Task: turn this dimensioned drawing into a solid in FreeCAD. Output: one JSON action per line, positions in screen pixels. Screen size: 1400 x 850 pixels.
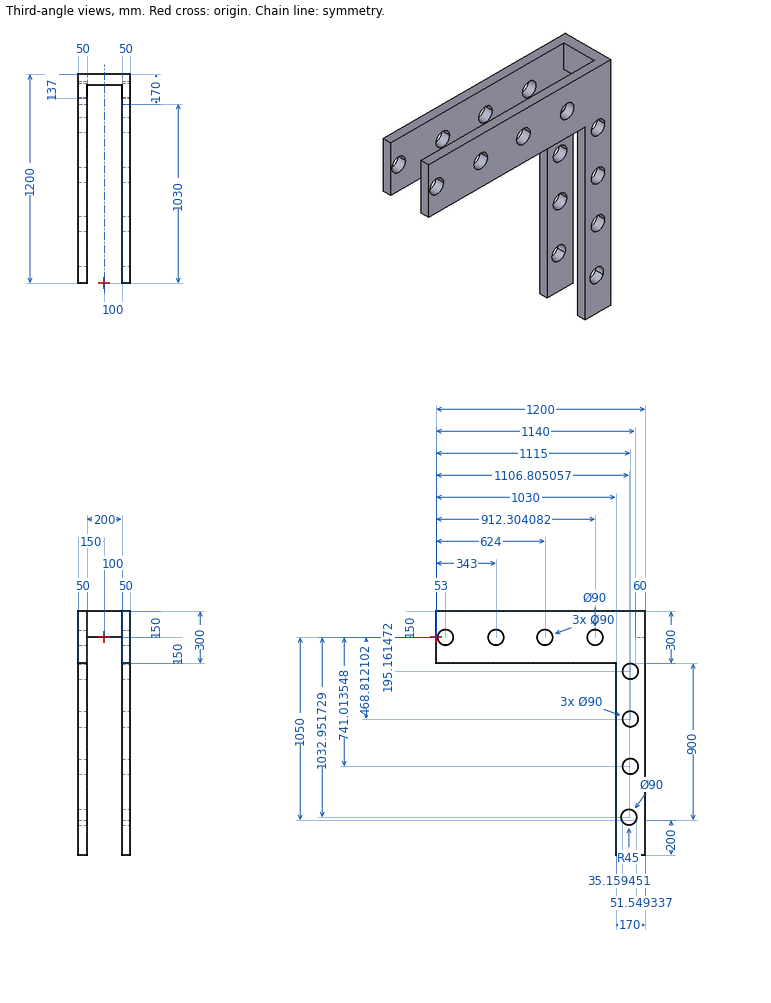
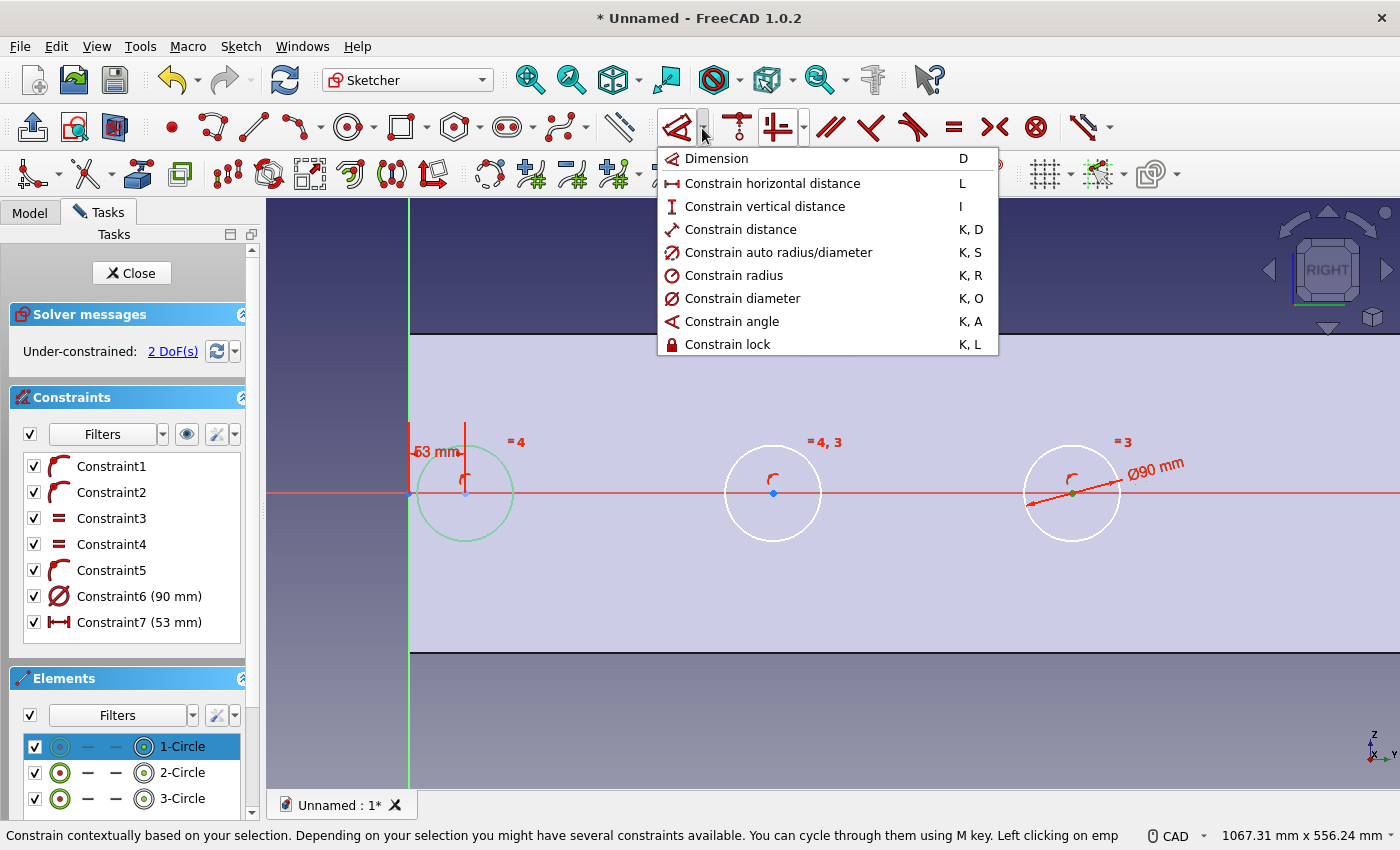
{"action": "left_click", "coordinate": [828, 184]}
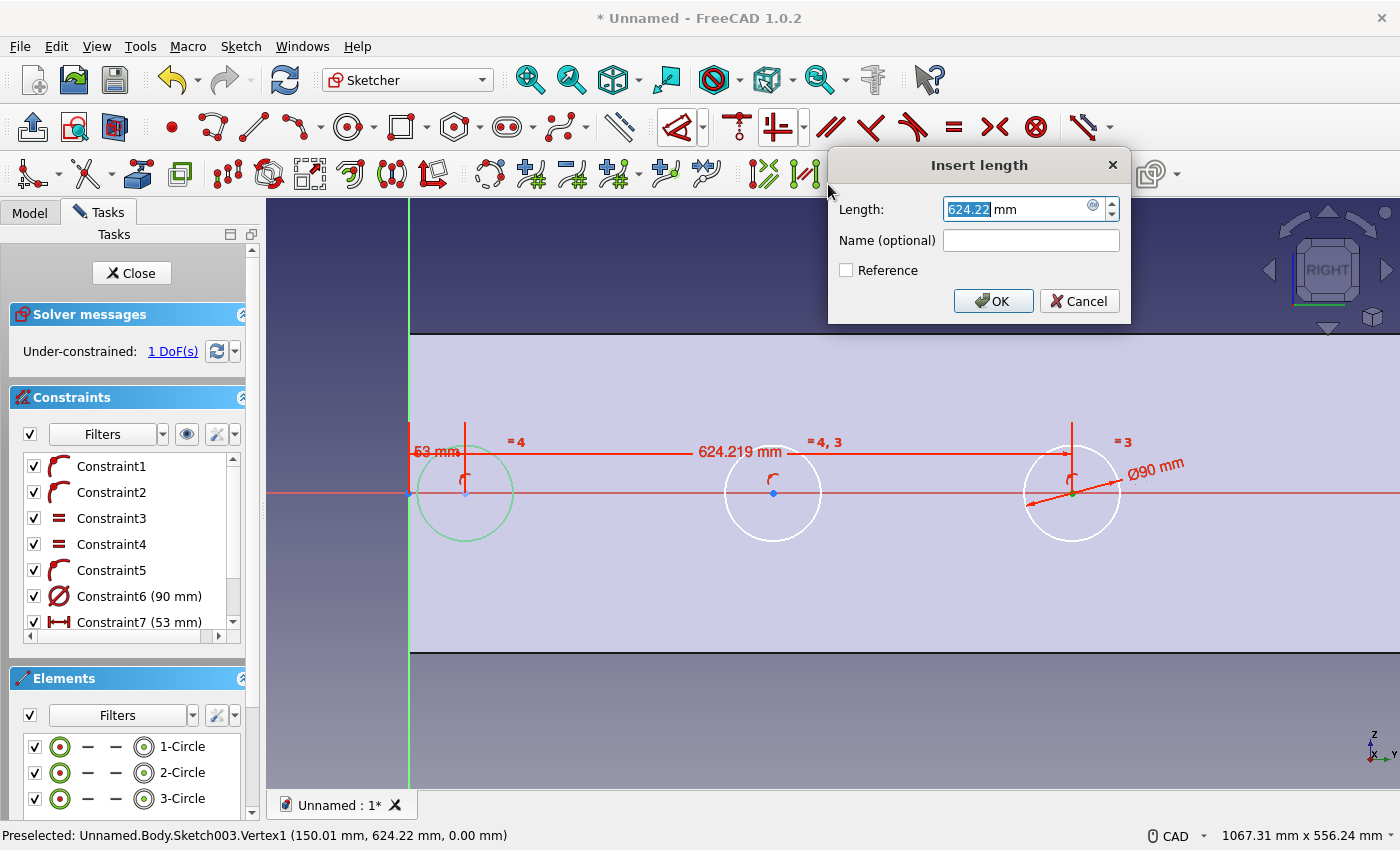
{"action": "type", "text": "624"}
{"action": "key", "text": "Return"}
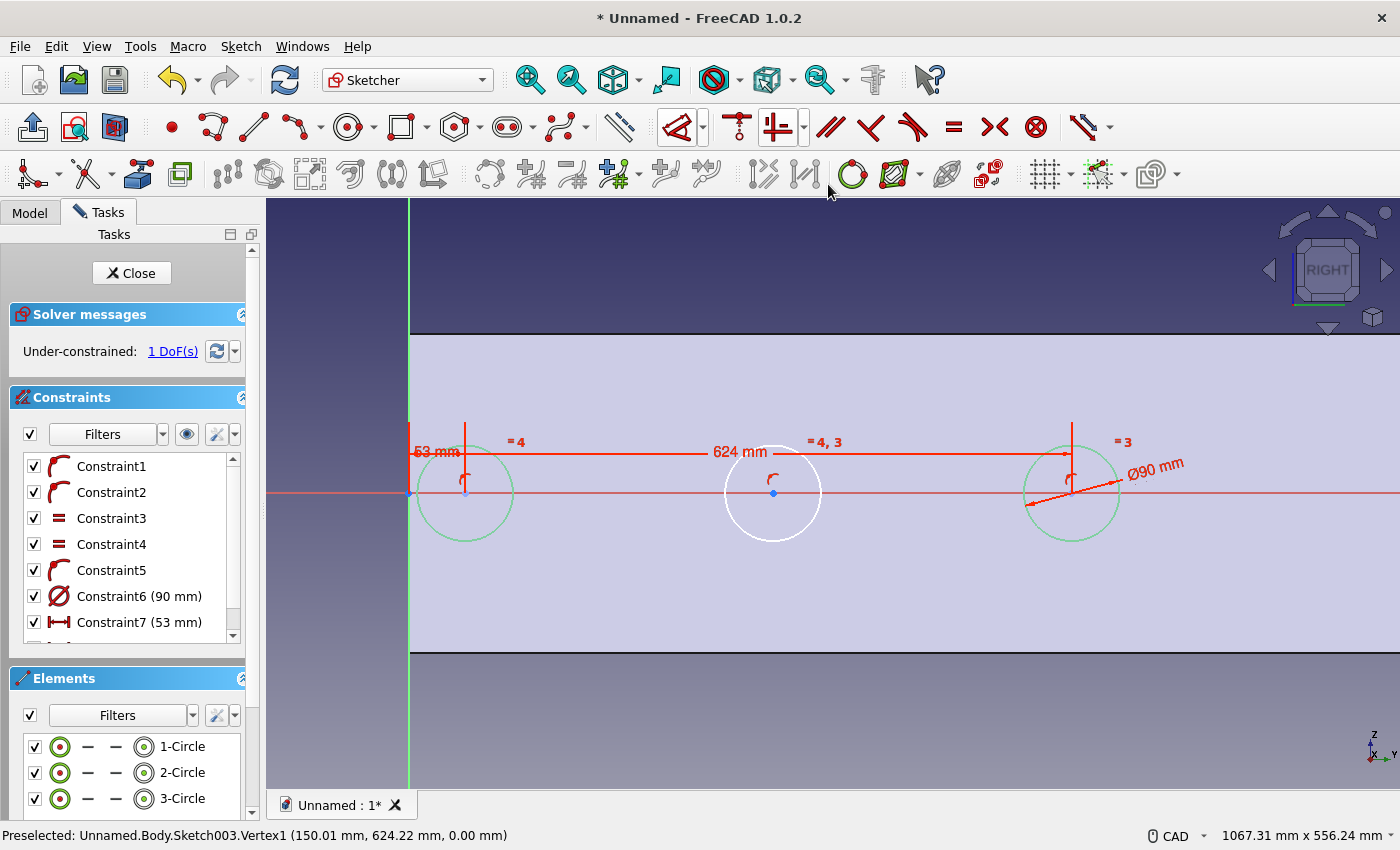
{"action": "left_click", "coordinate": [773, 493]}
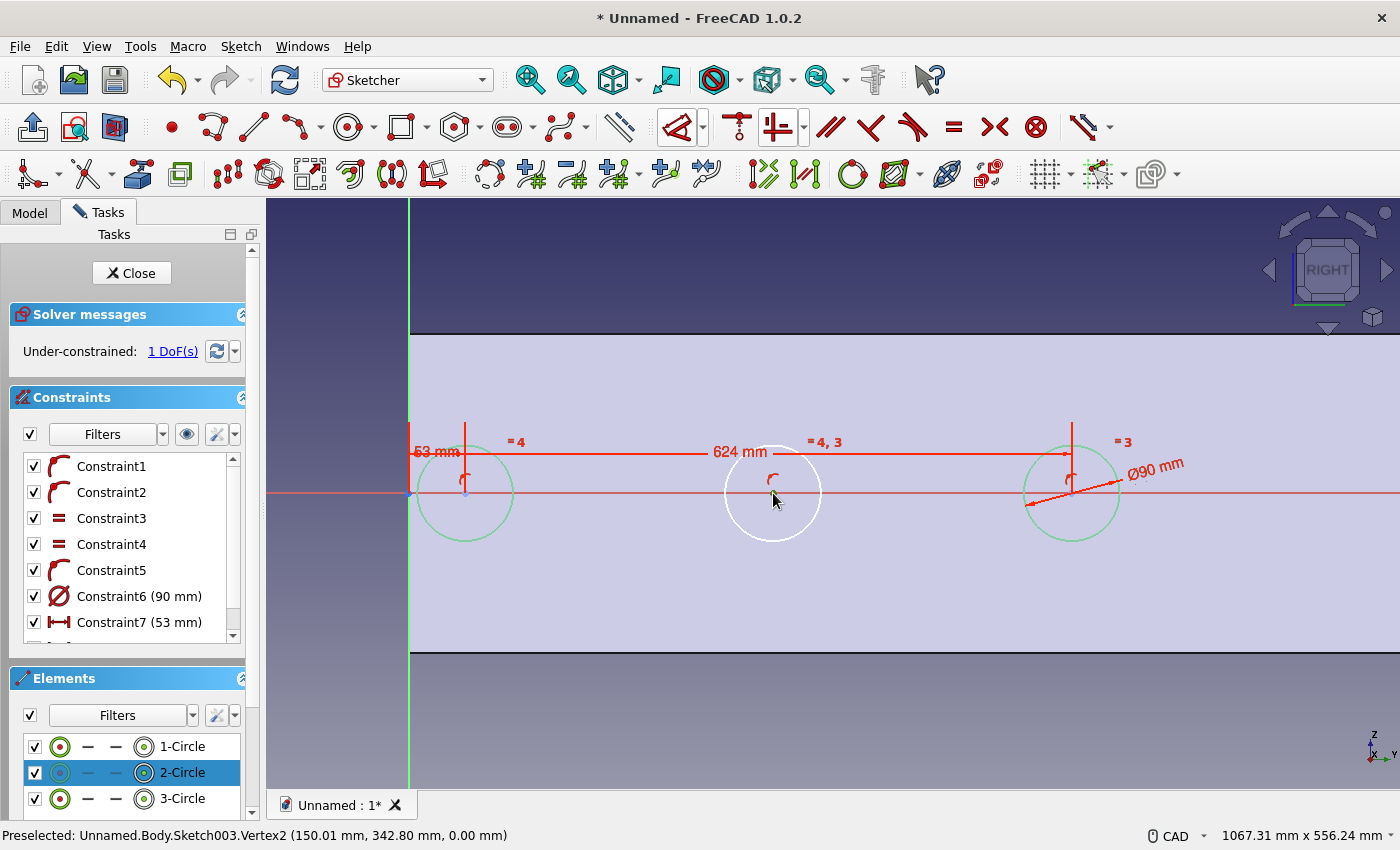
{"action": "left_click", "coordinate": [702, 128]}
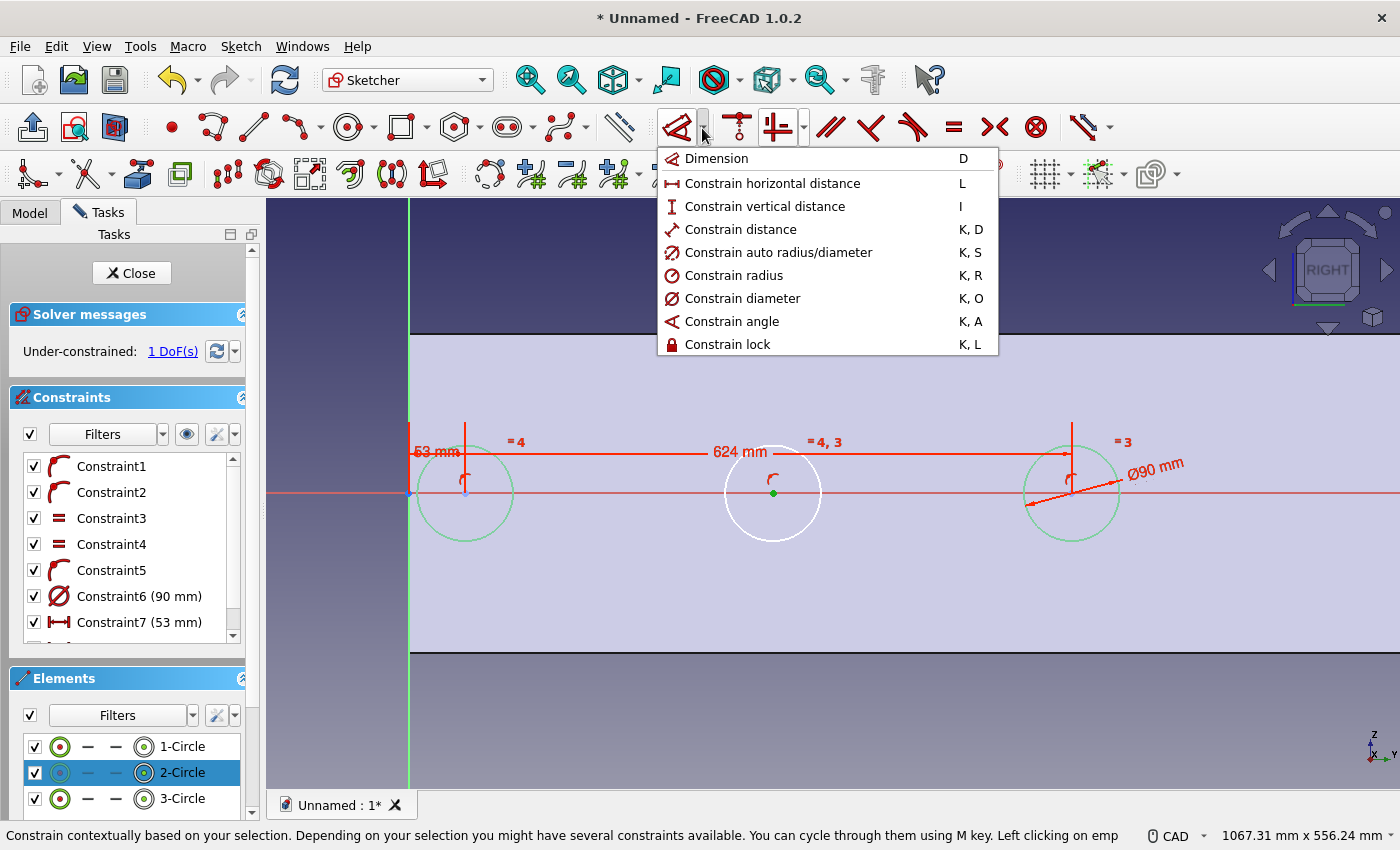
{"action": "left_click", "coordinate": [828, 184]}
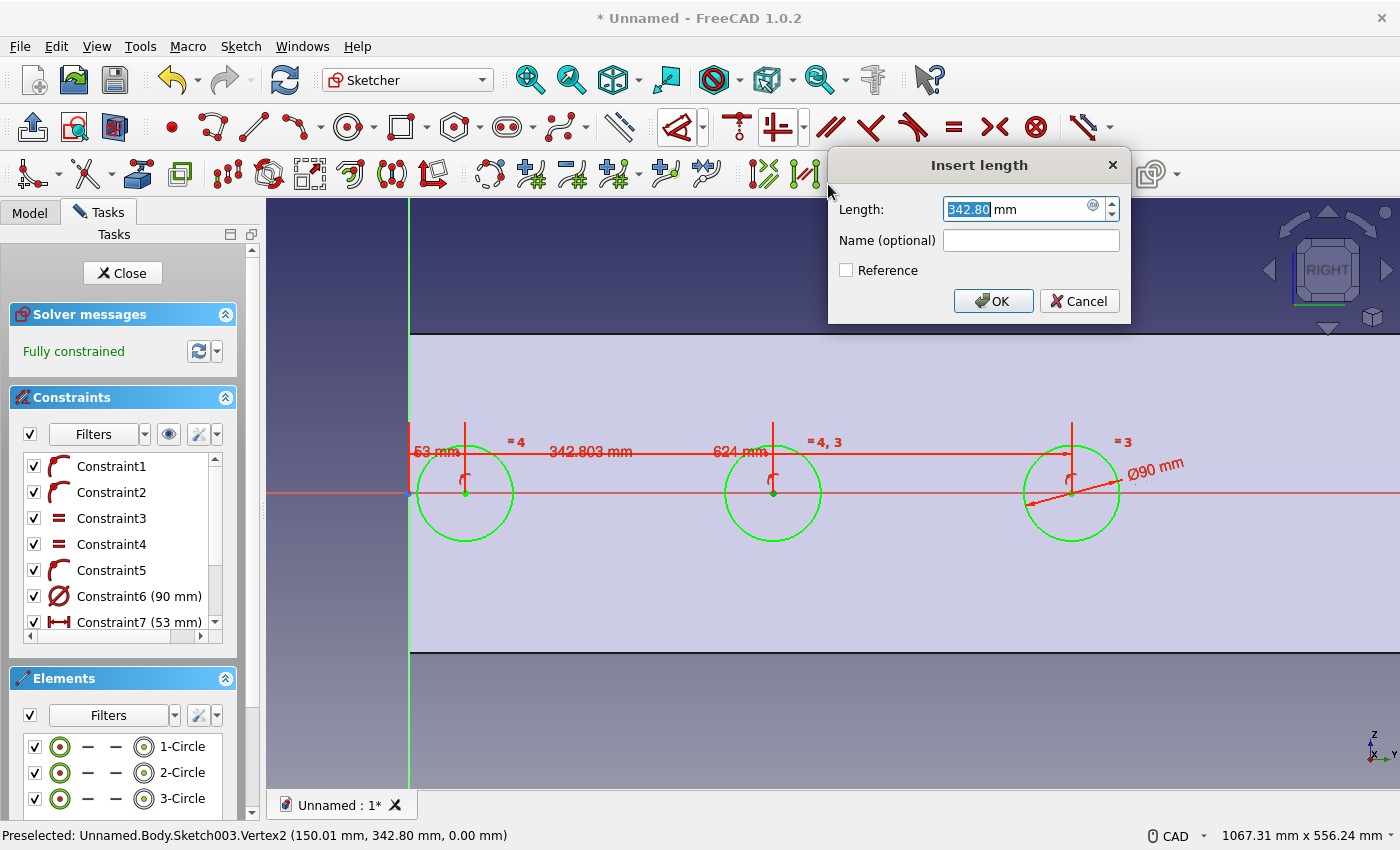
{"action": "type", "text": "343"}
{"action": "key", "text": "Return"}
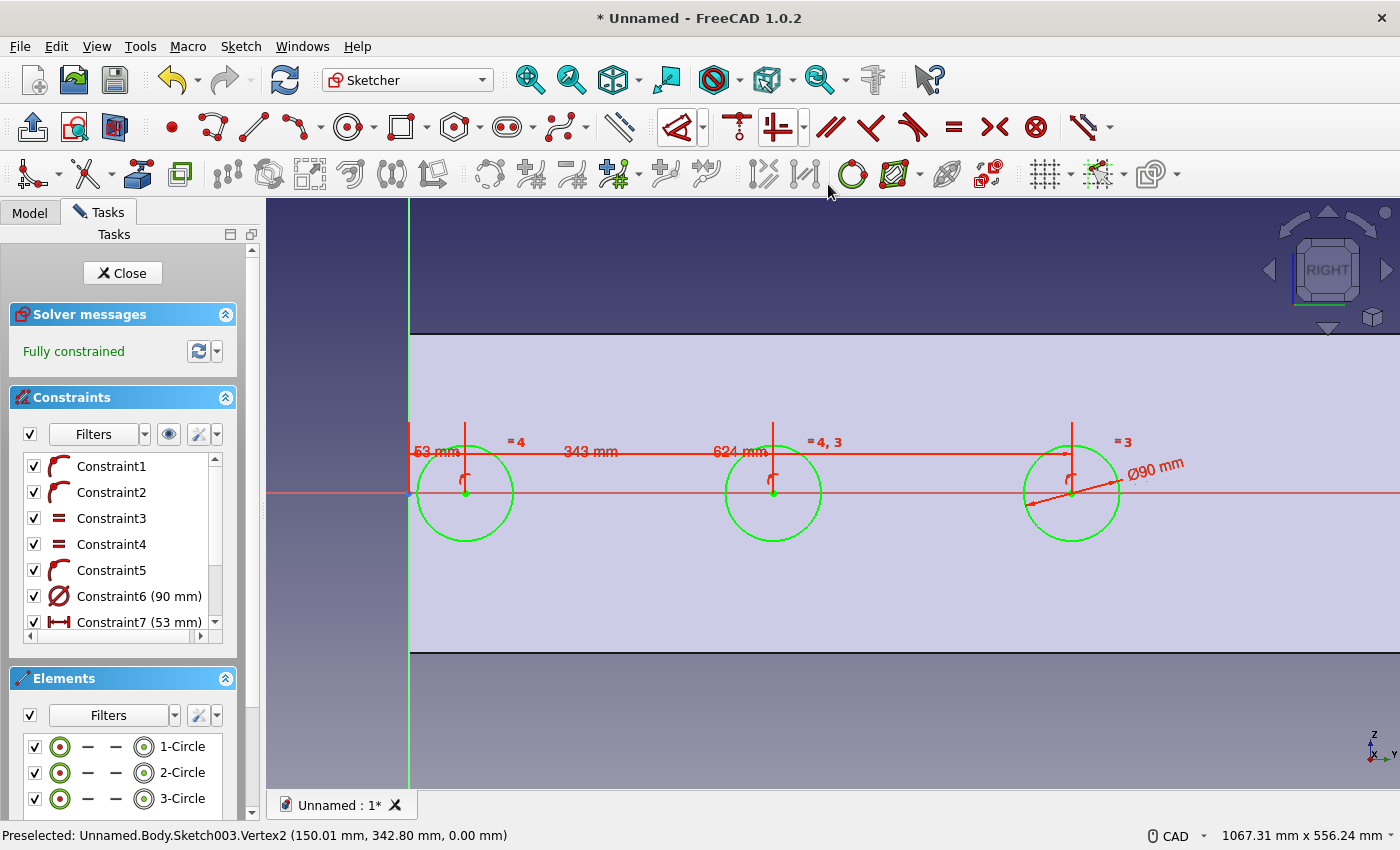
{"action": "left_click", "coordinate": [123, 273]}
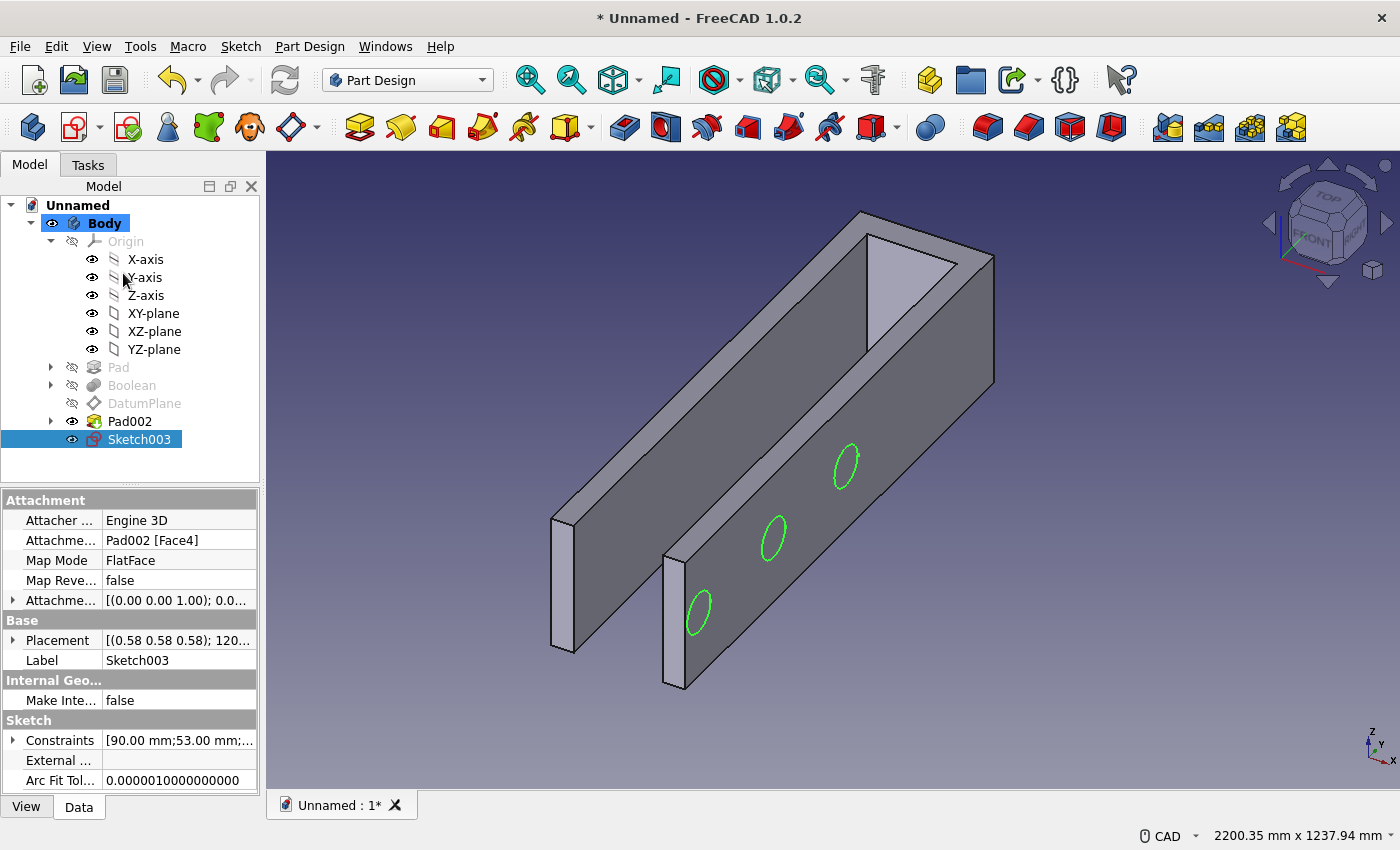
{"action": "left_click", "coordinate": [625, 128]}